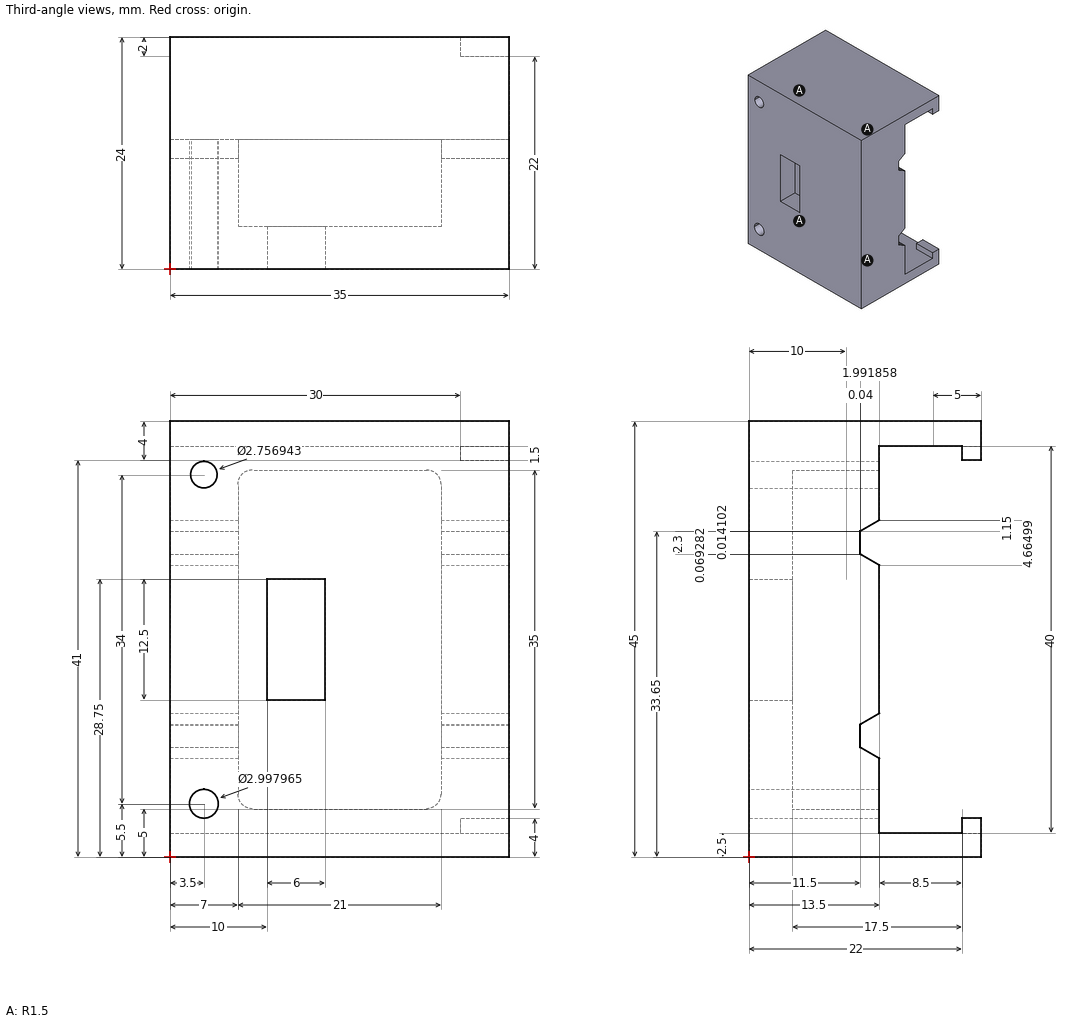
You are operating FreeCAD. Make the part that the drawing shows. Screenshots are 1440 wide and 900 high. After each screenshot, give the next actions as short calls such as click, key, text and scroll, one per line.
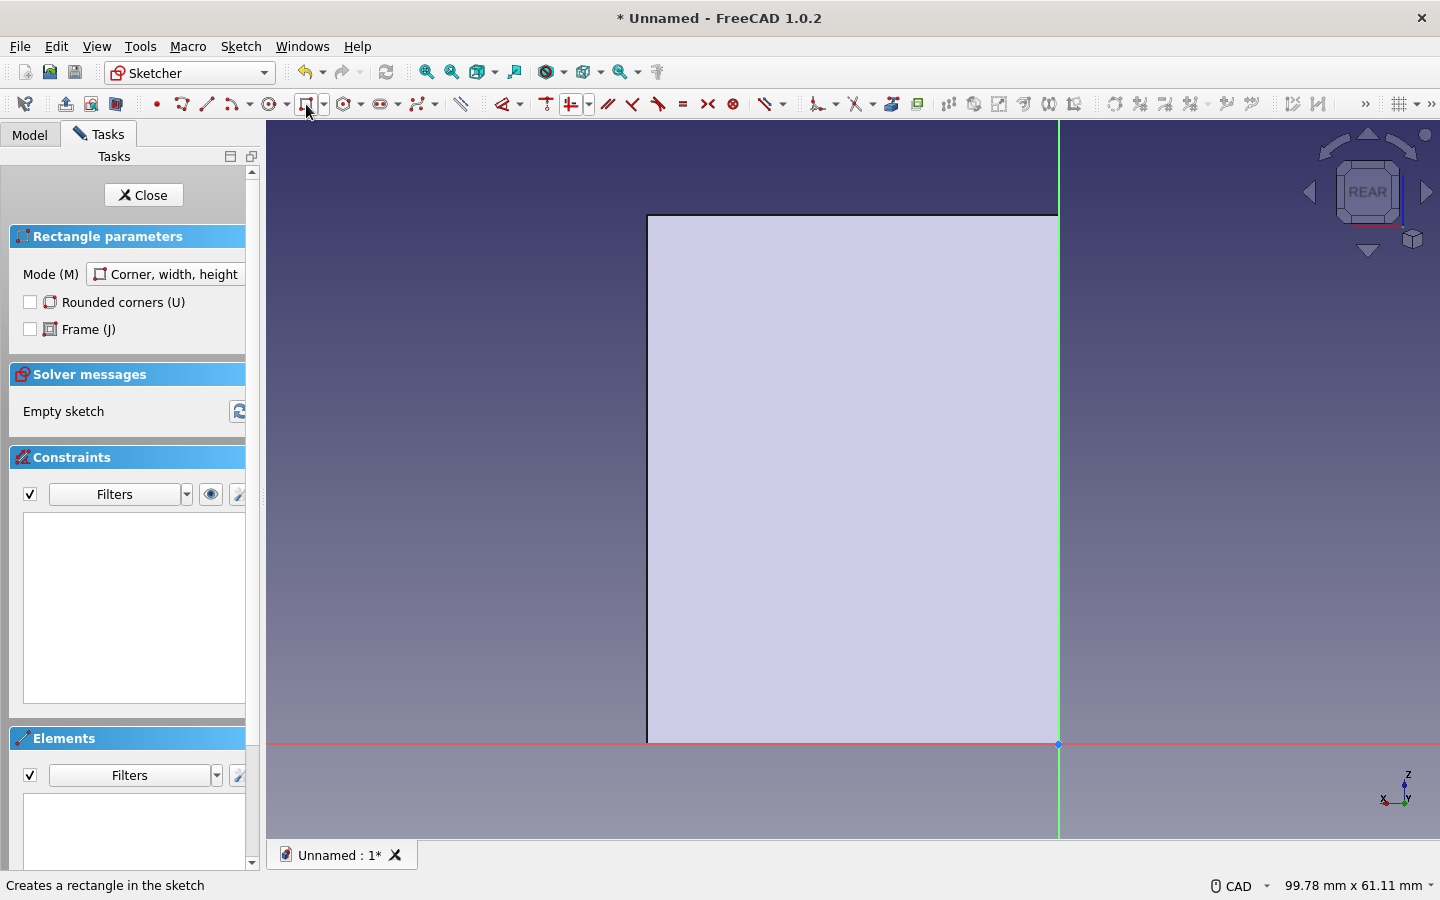
click(729, 274)
click(977, 685)
key(Escape)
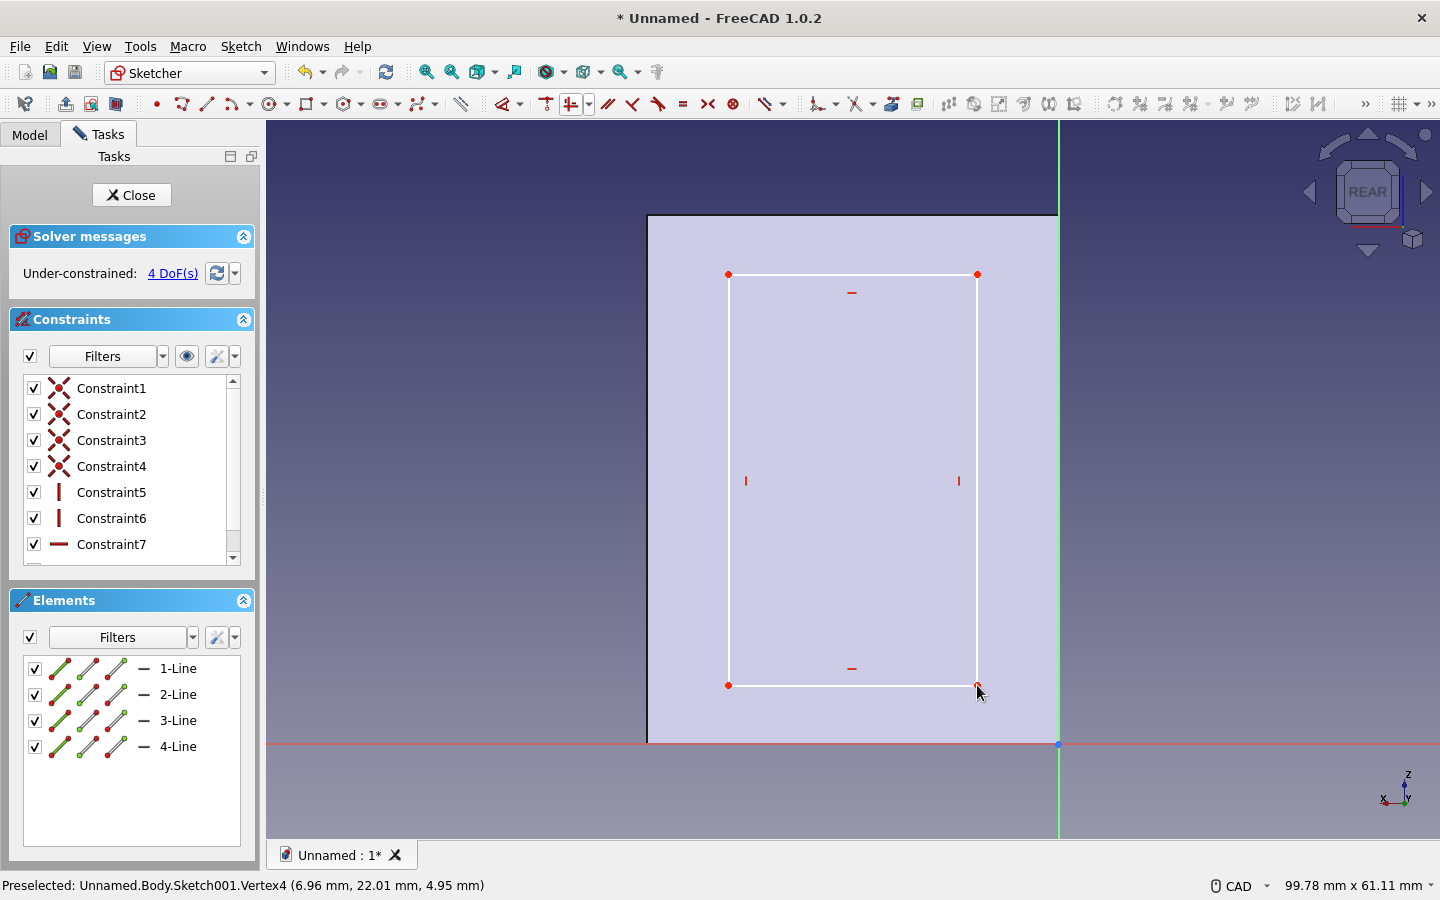
key(d)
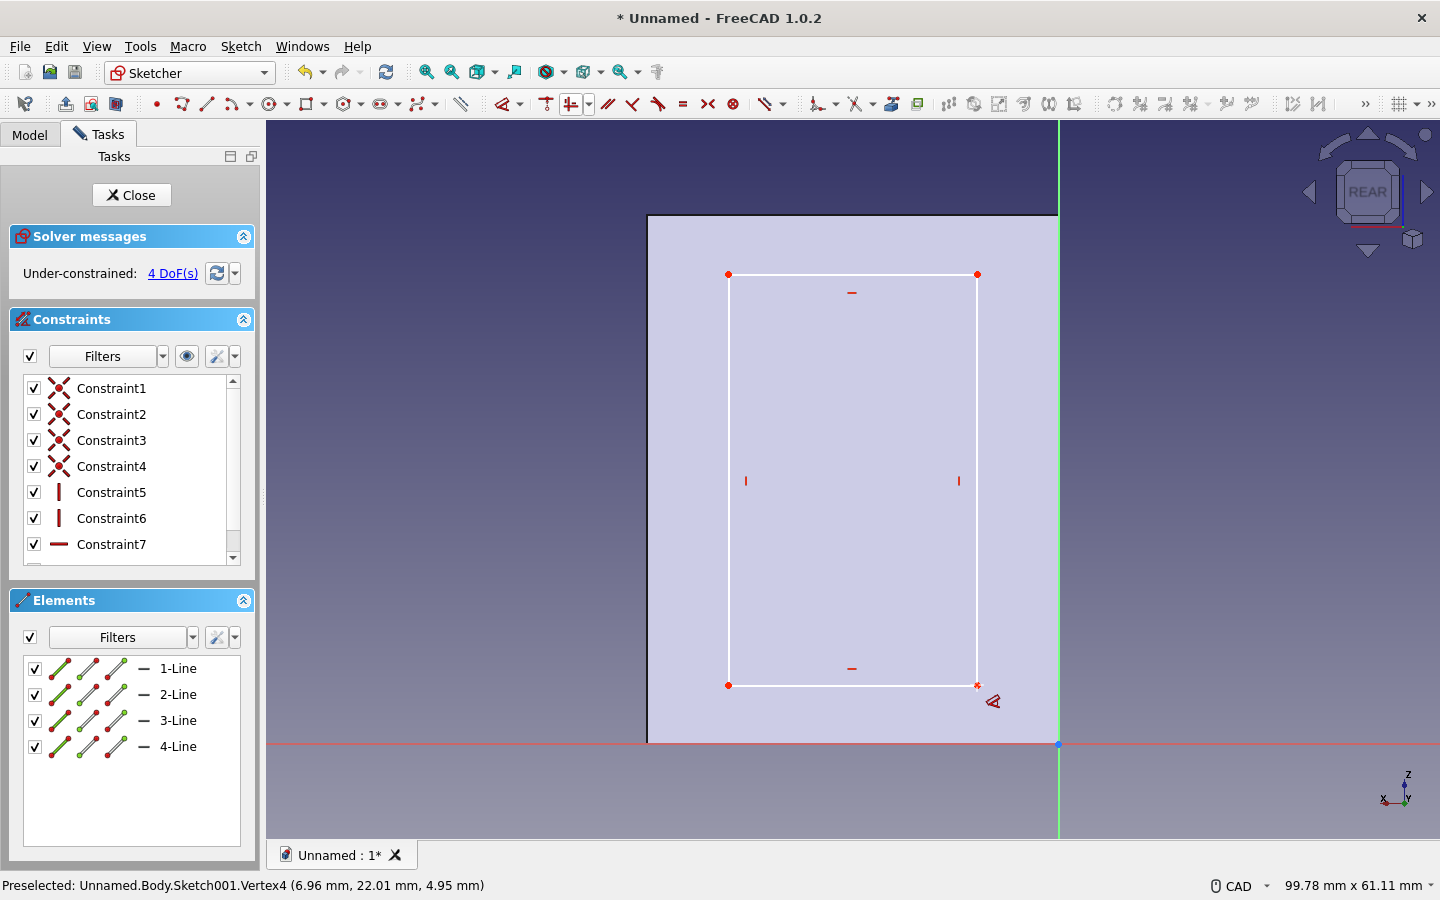
click(729, 398)
click(695, 480)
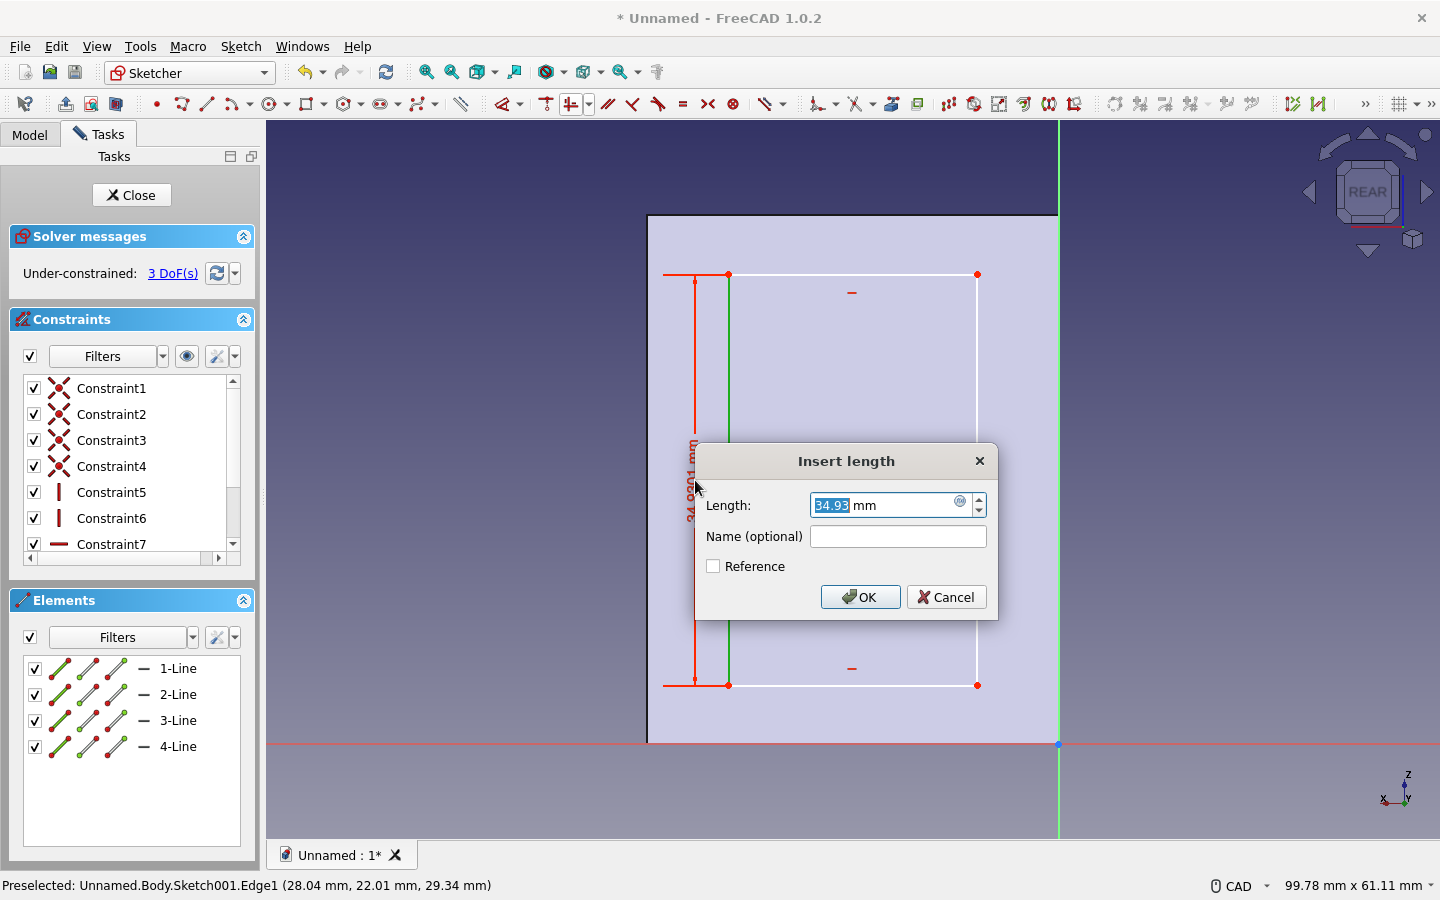
text(35)
key(Return)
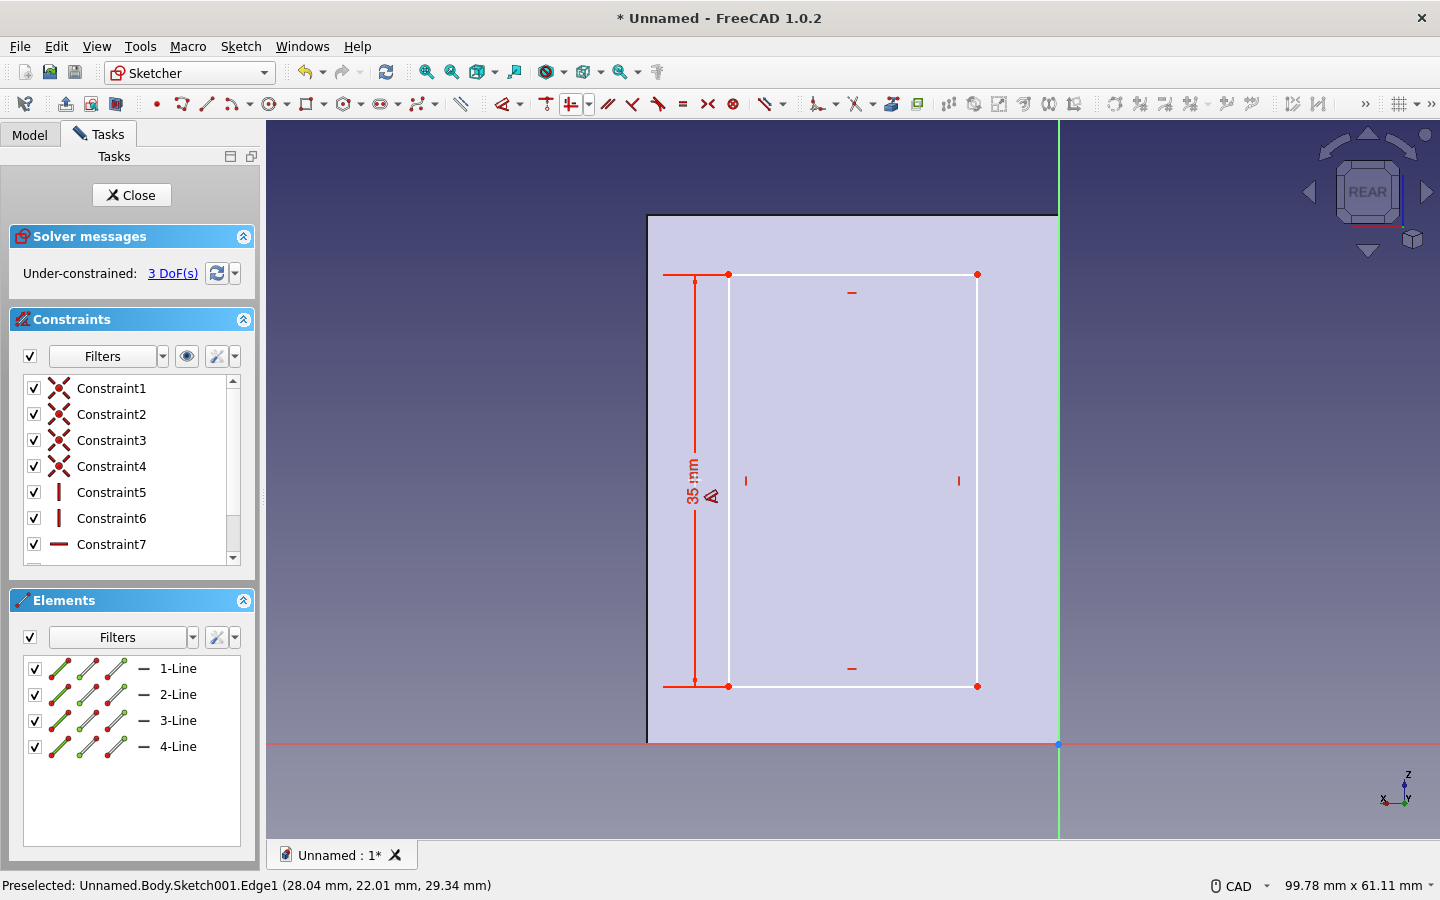
click(803, 687)
click(853, 721)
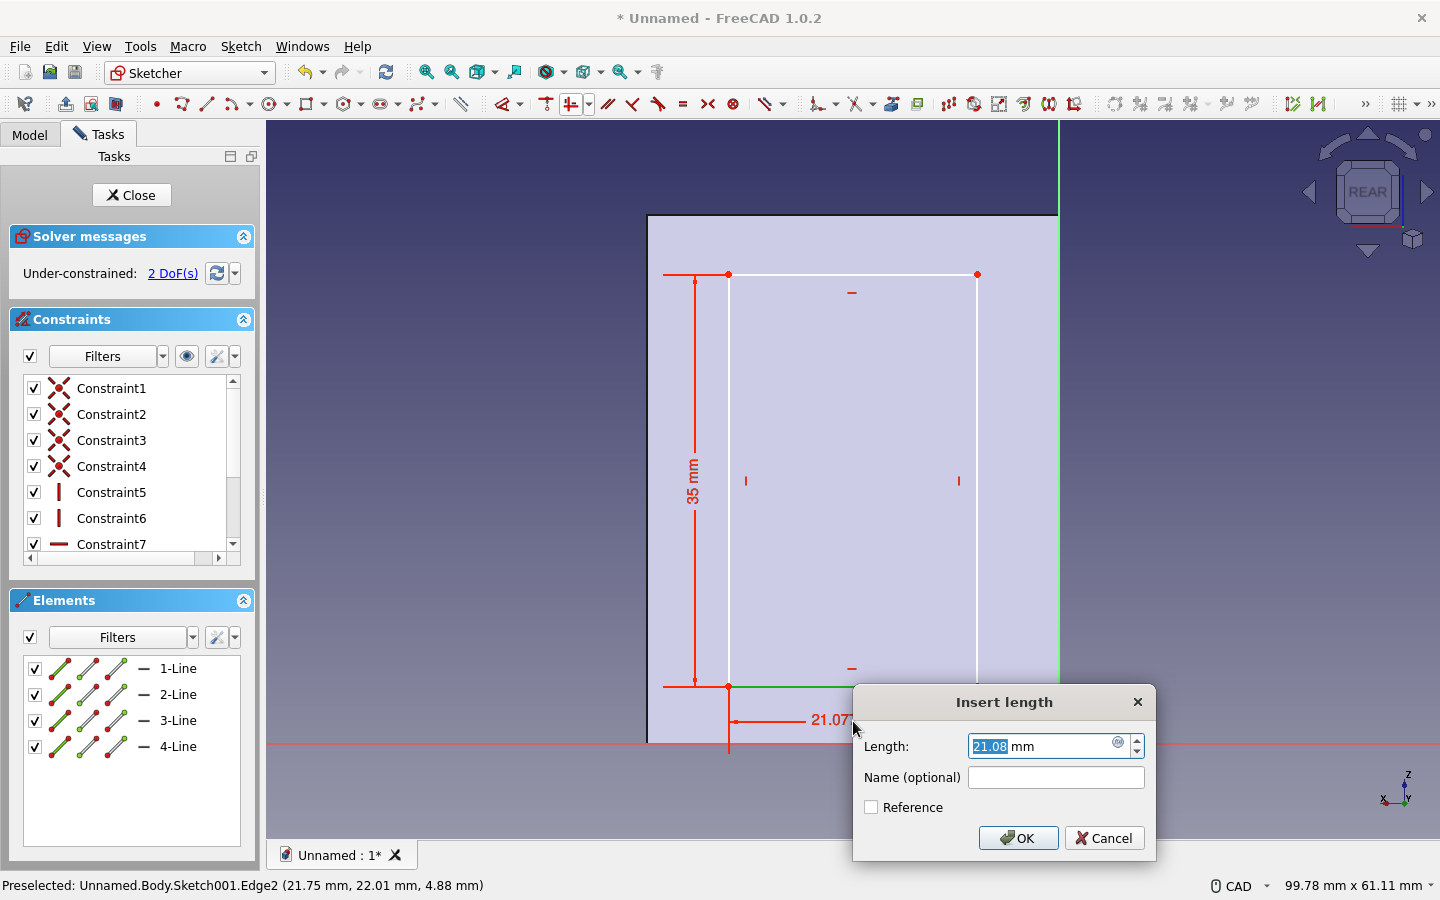
text(21)
key(Return)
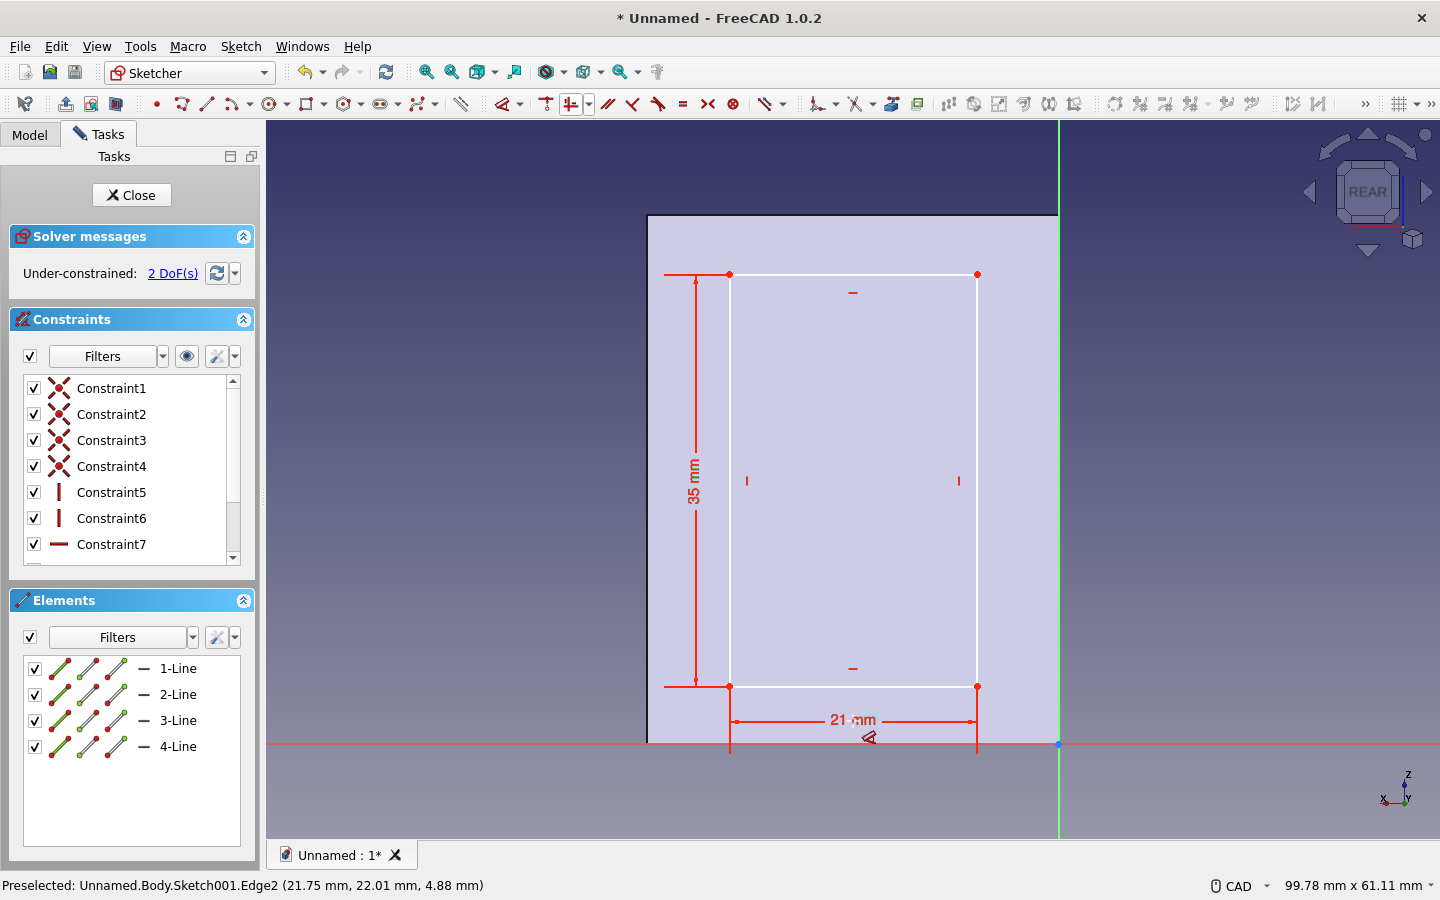
click(730, 687)
click(1093, 716)